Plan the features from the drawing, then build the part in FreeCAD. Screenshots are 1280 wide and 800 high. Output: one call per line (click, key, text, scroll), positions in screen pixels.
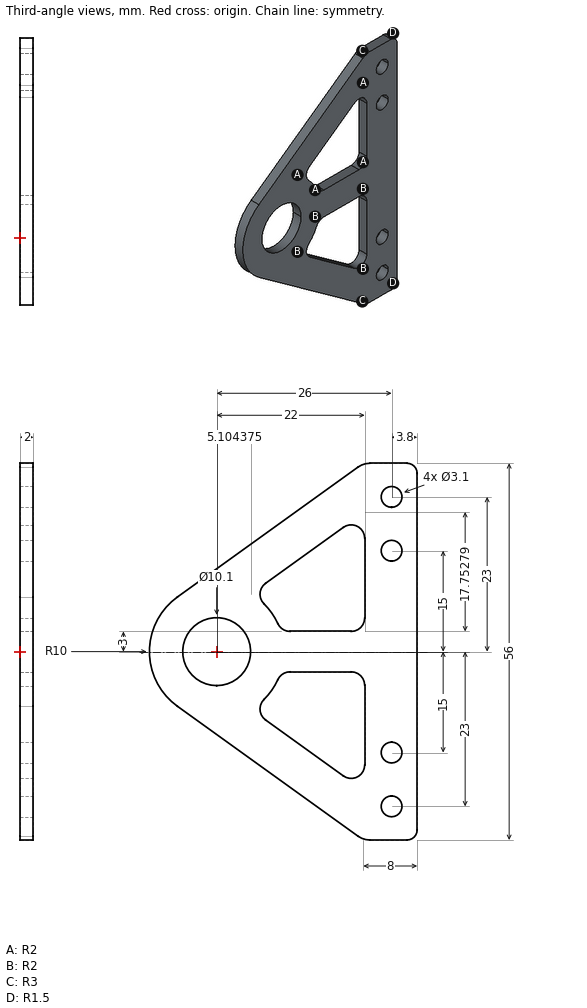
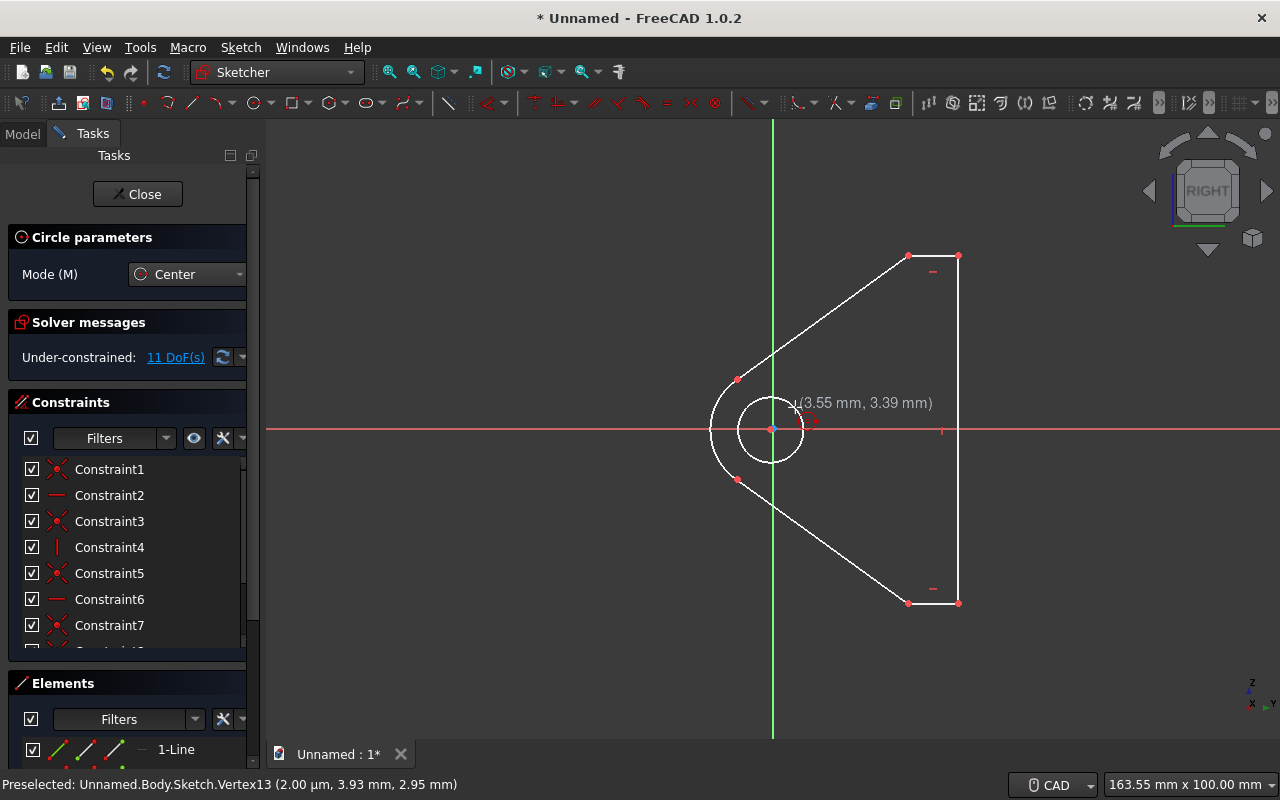
scroll(934, 286, up, 5)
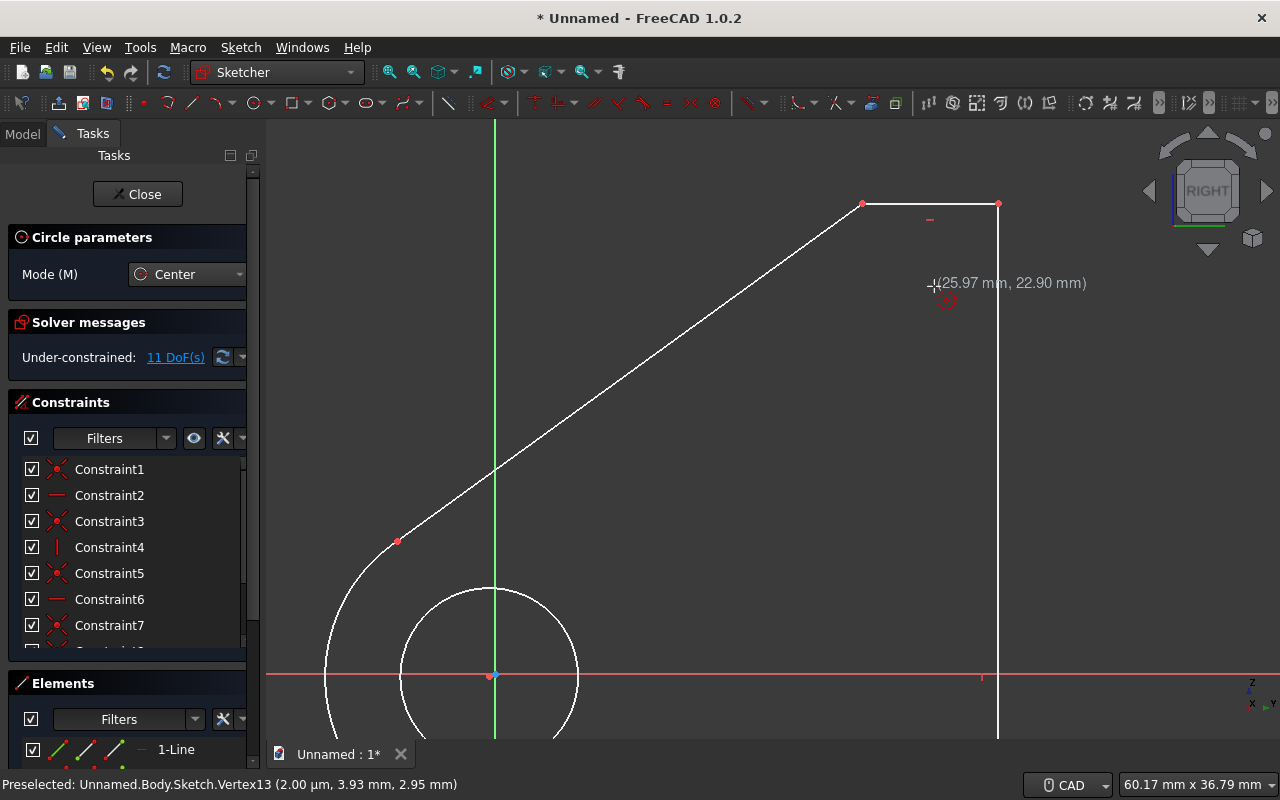
click(933, 287)
click(952, 268)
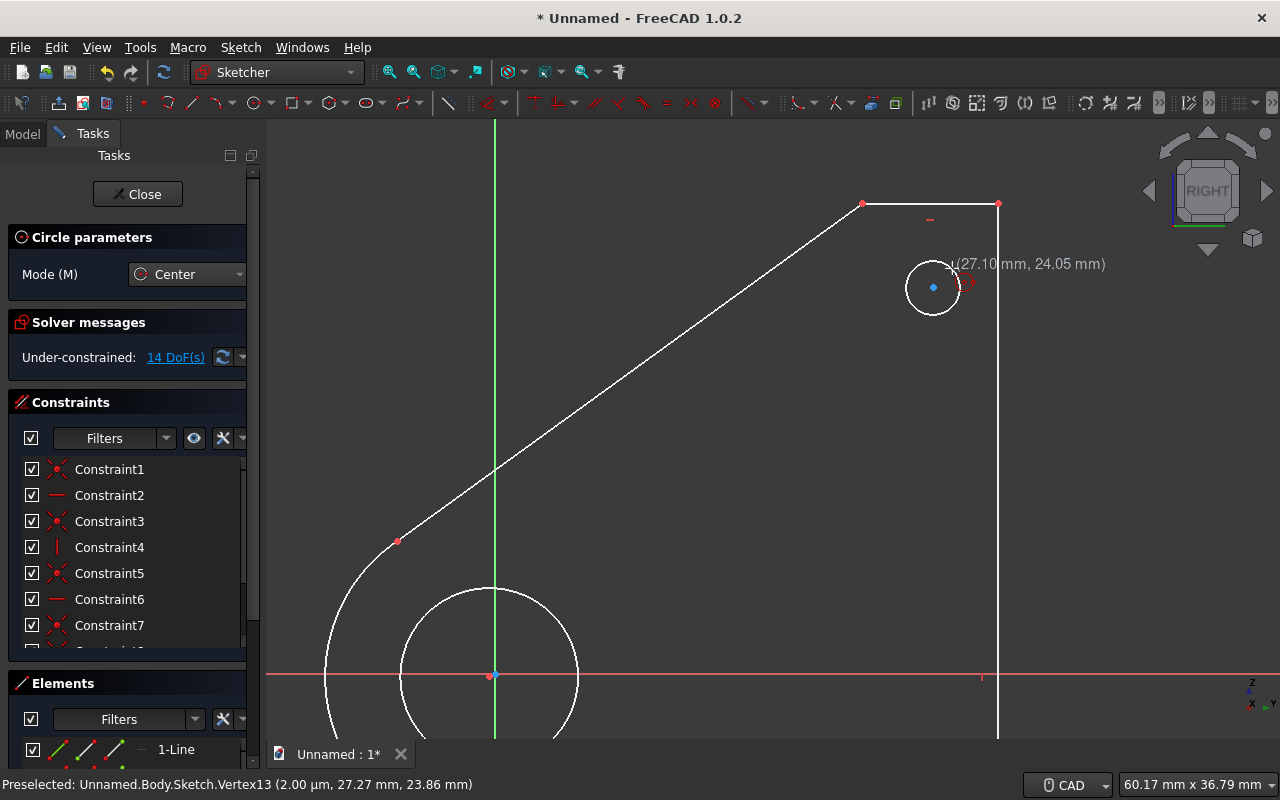
click(933, 421)
click(952, 403)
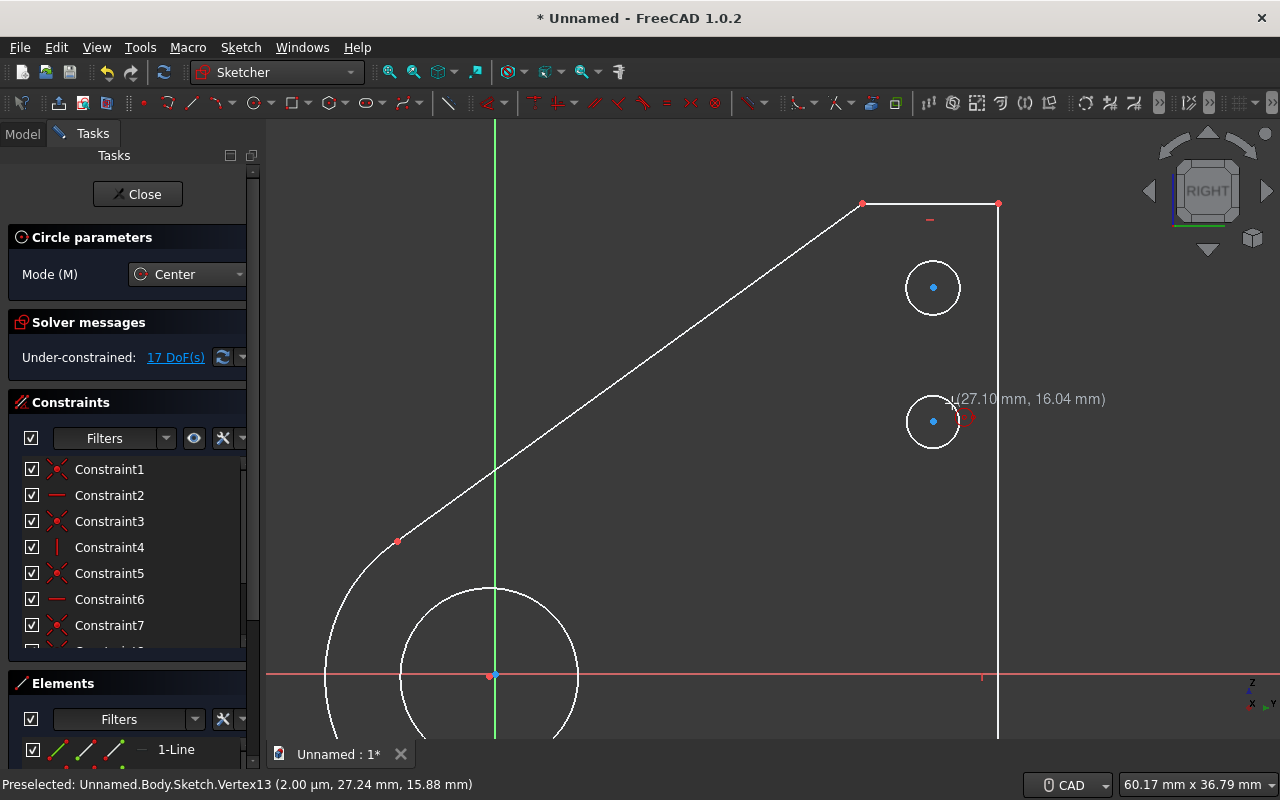
scroll(739, 229, down, 4)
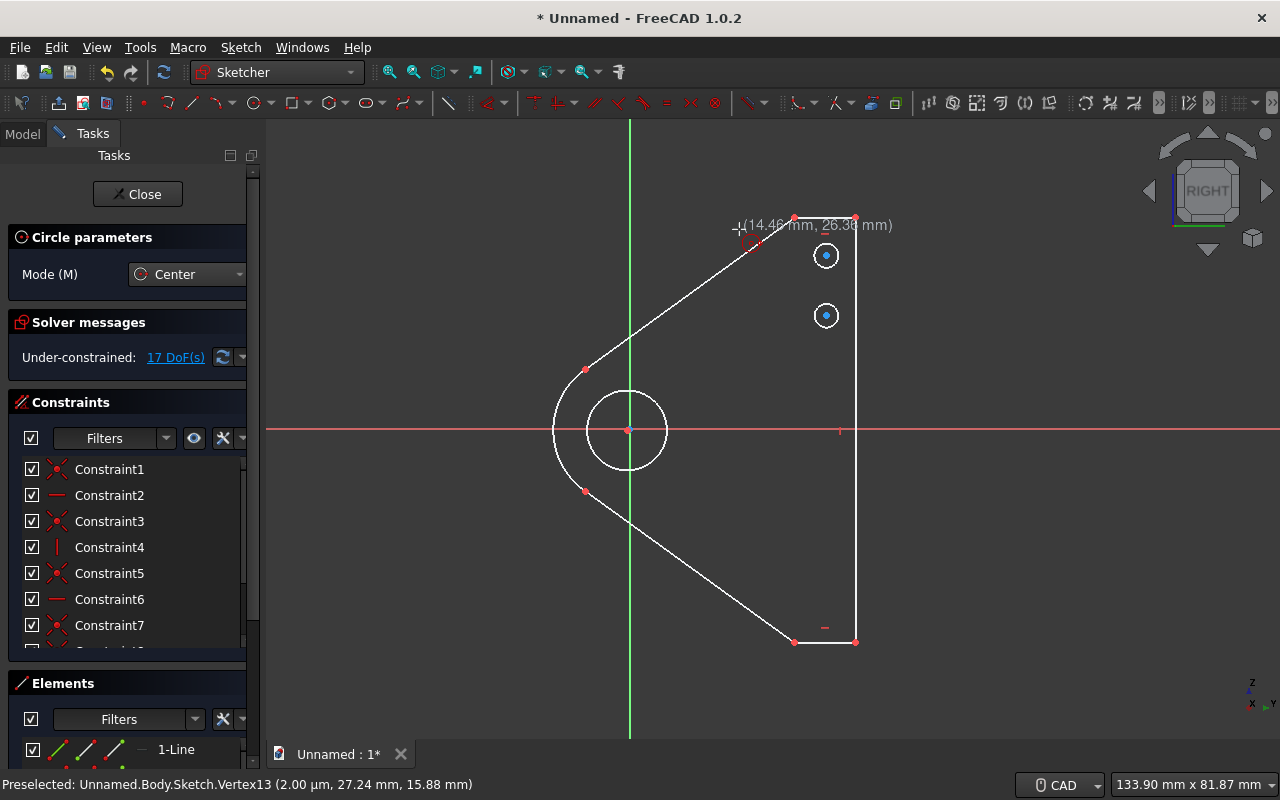
scroll(827, 543, up, 4)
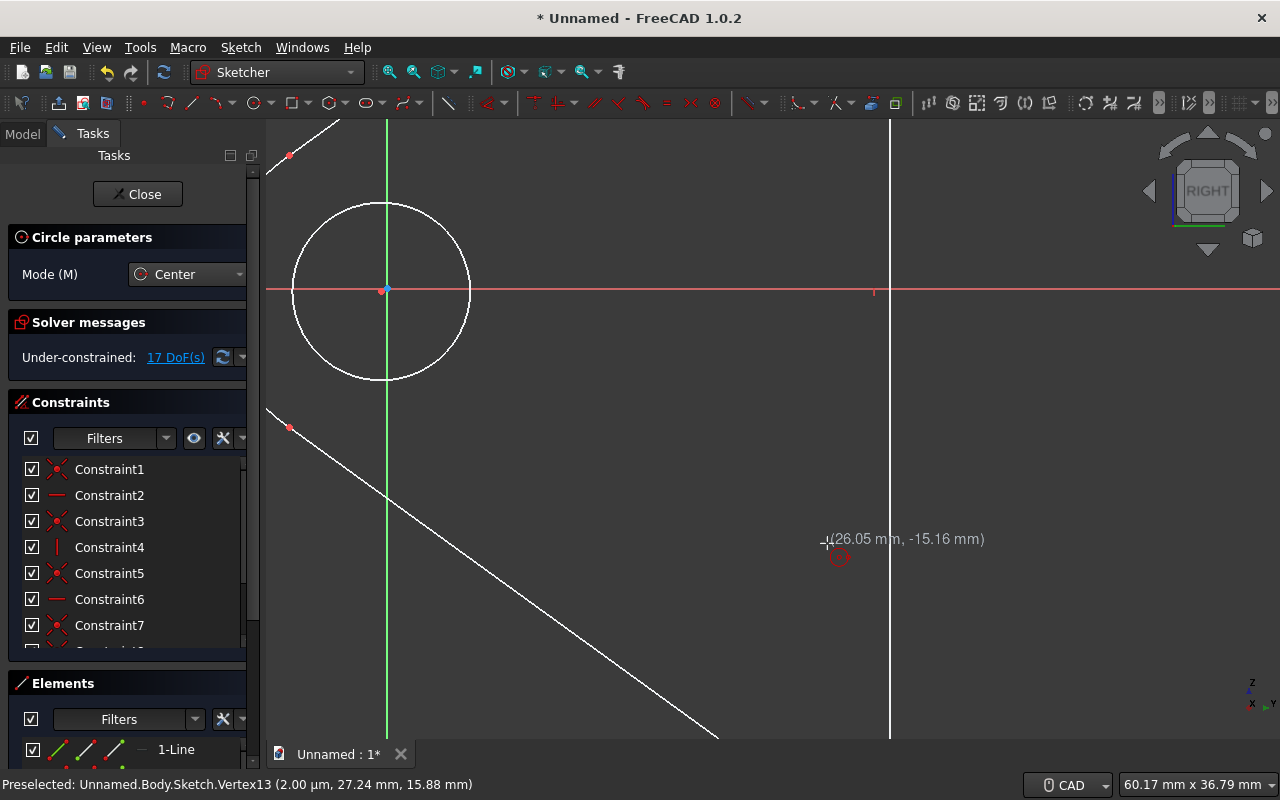
click(825, 542)
click(844, 523)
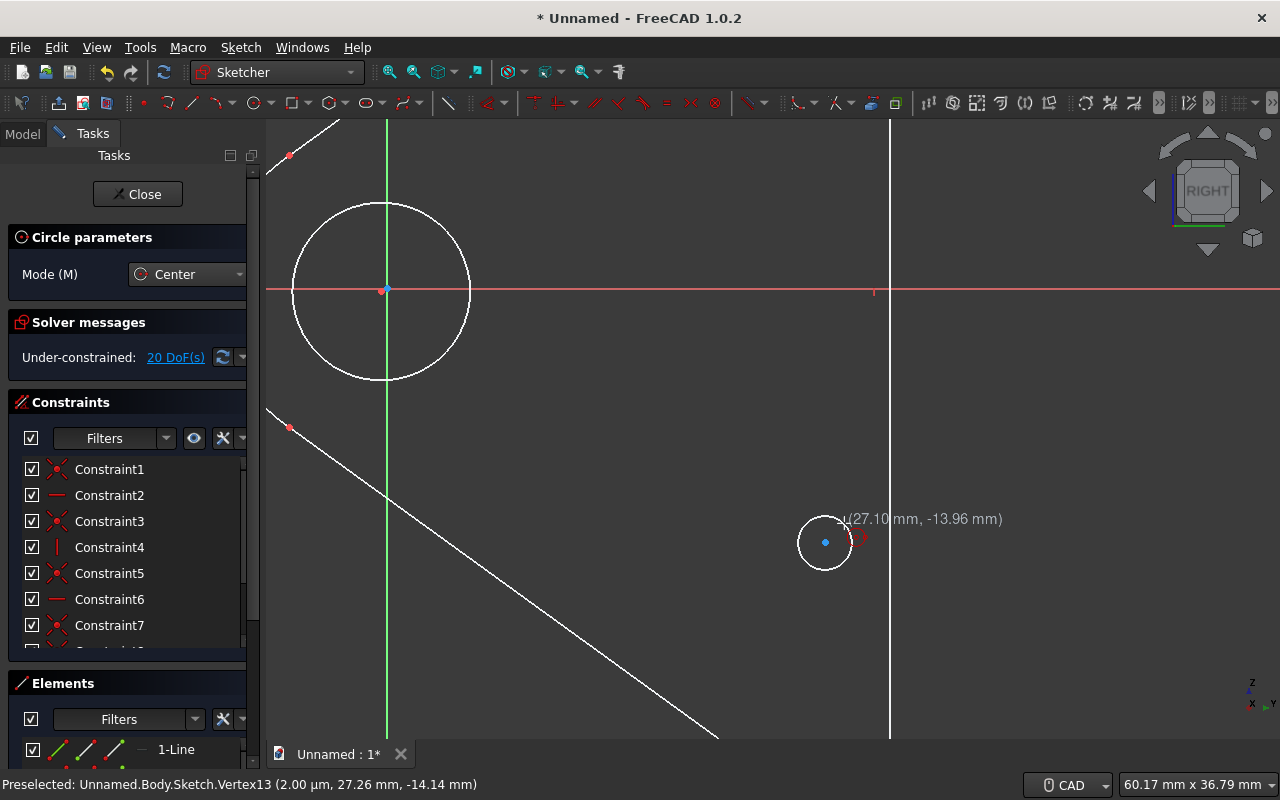
click(825, 676)
click(844, 658)
key(Escape)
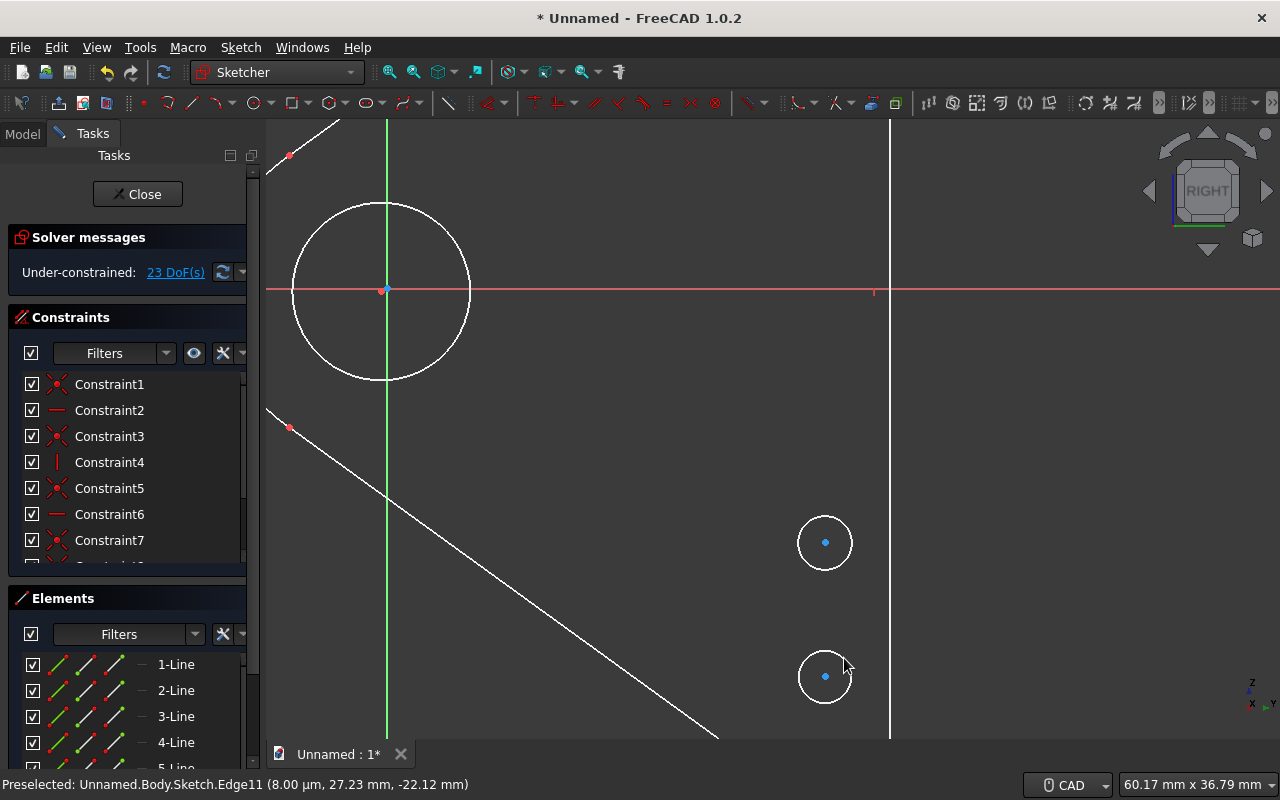
click(429, 529)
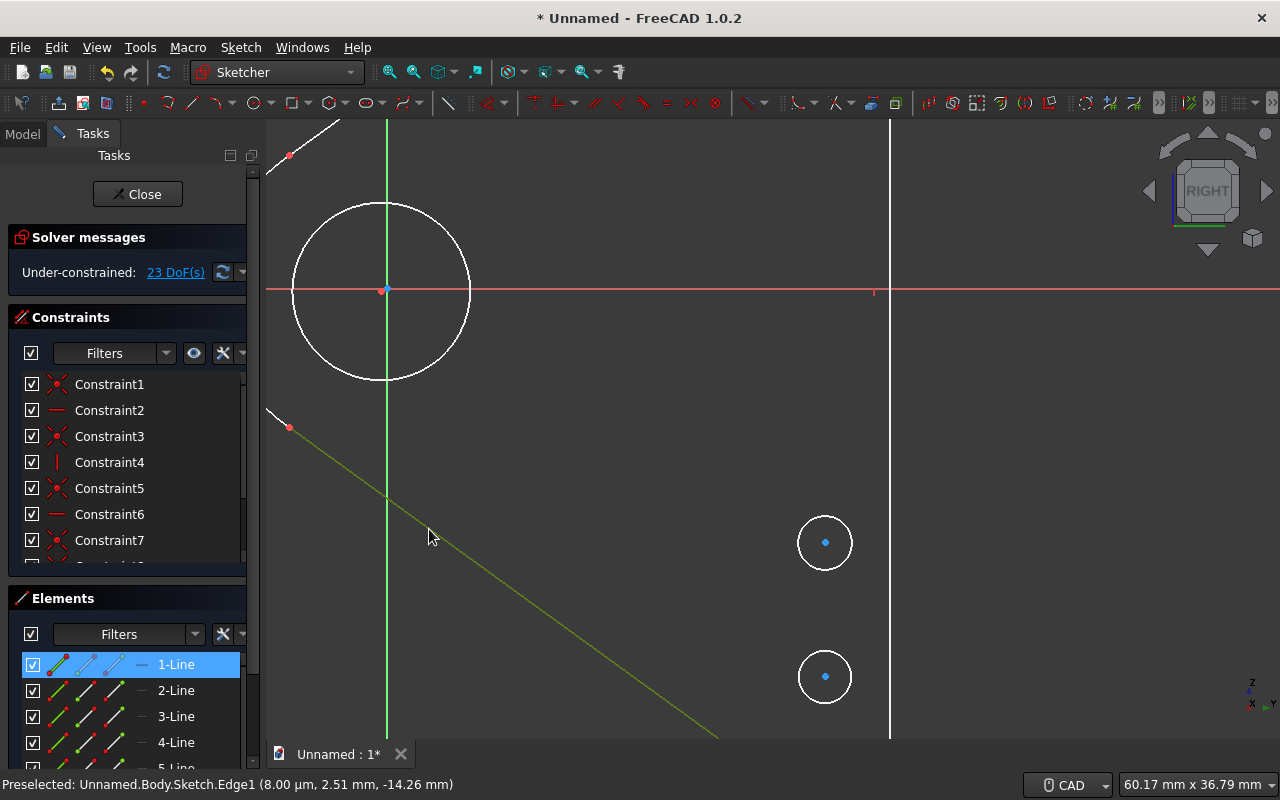
scroll(827, 543, down, 4)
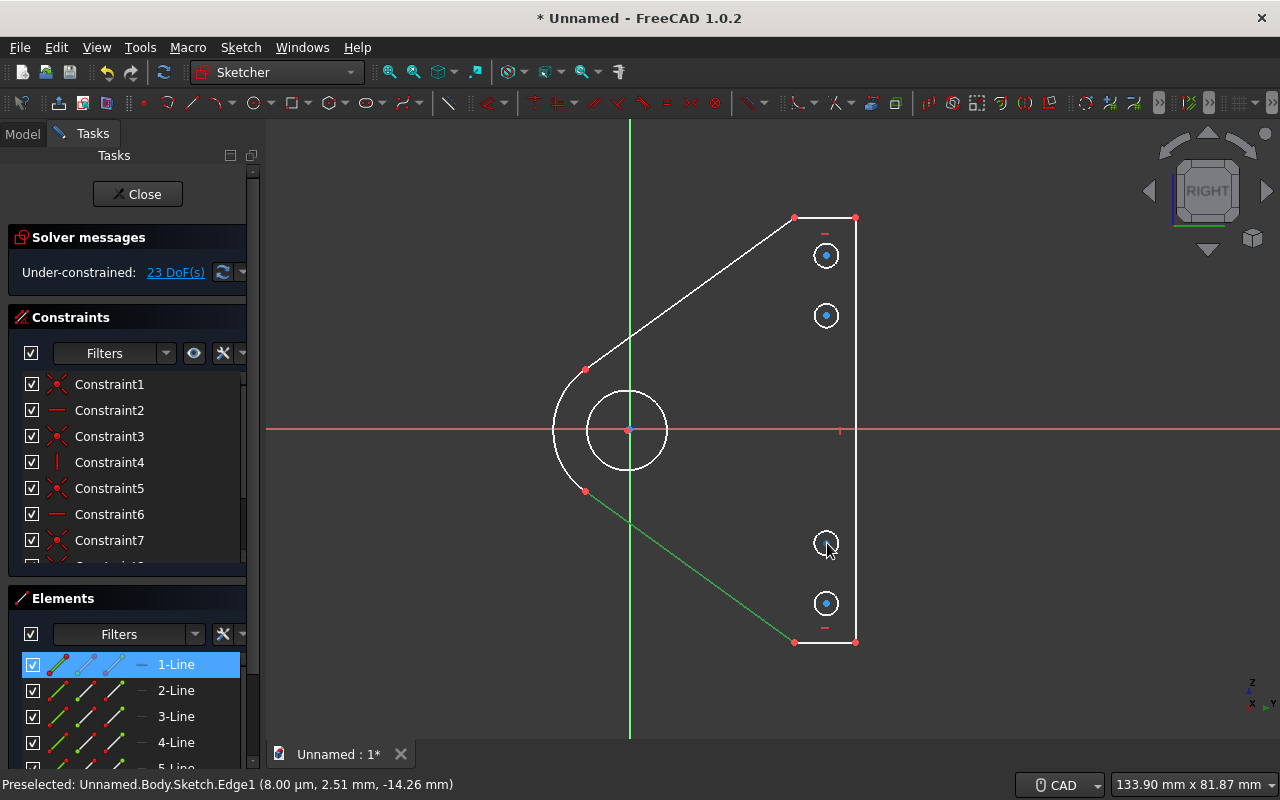
click(559, 402)